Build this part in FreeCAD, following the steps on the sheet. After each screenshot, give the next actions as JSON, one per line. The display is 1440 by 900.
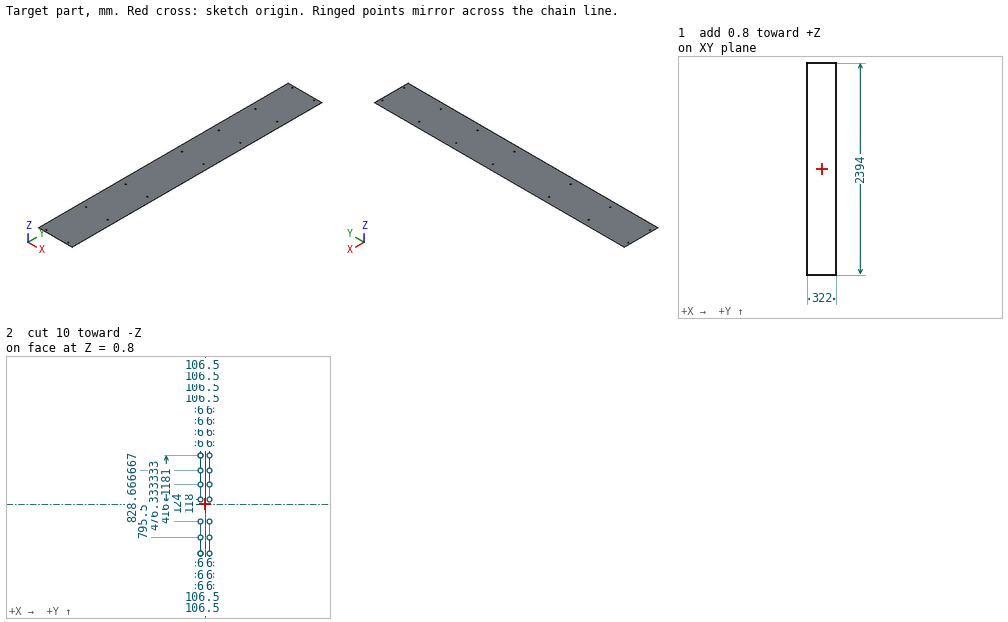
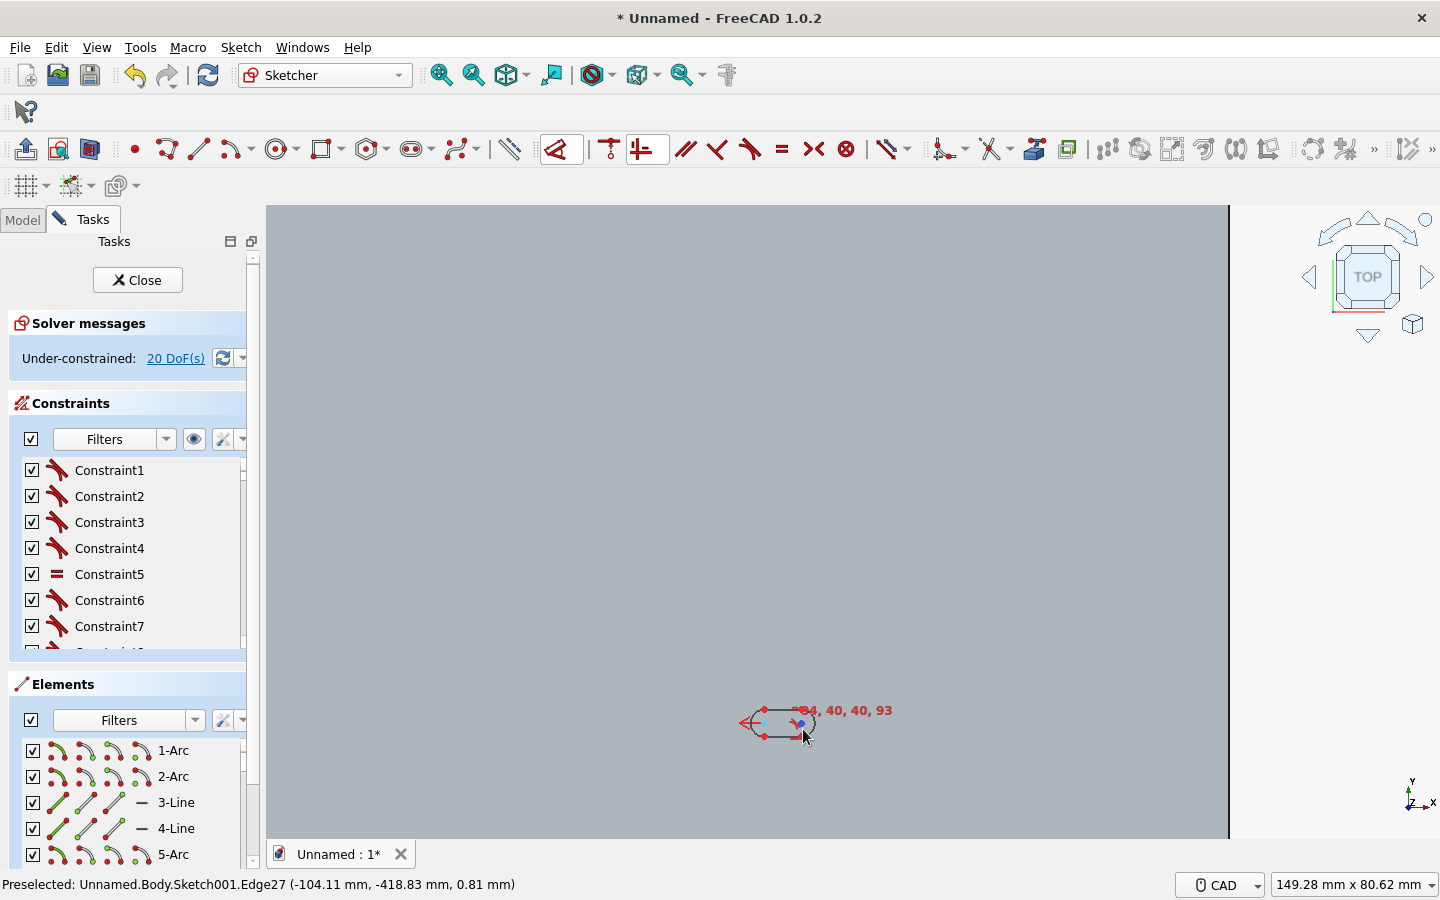
{"action": "left_click", "coordinate": [775, 710]}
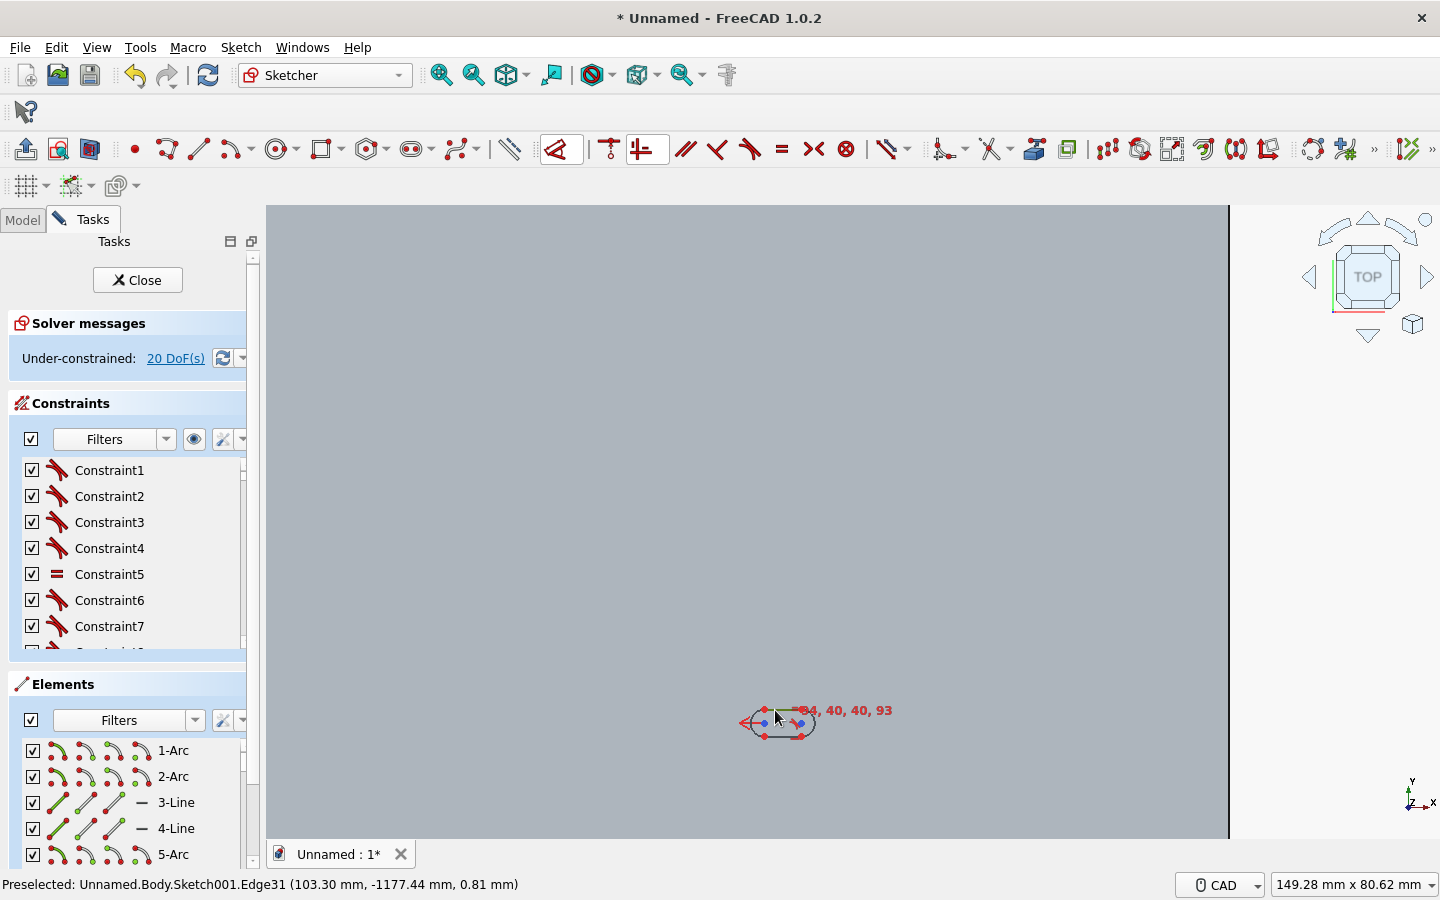
{"action": "key", "text": "l"}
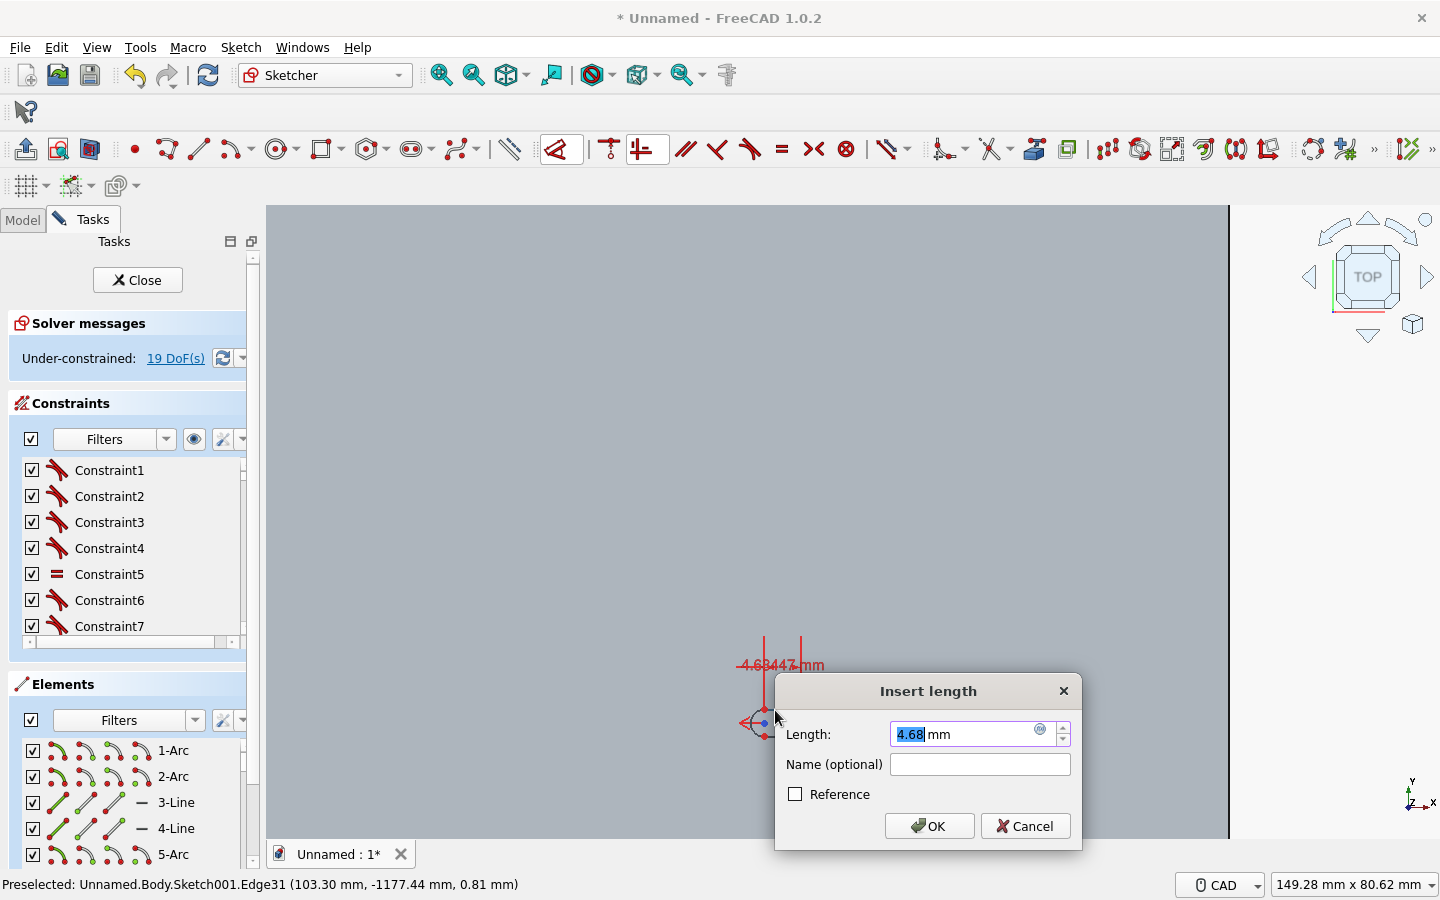
{"action": "type", "text": "6"}
{"action": "key", "text": "Return"}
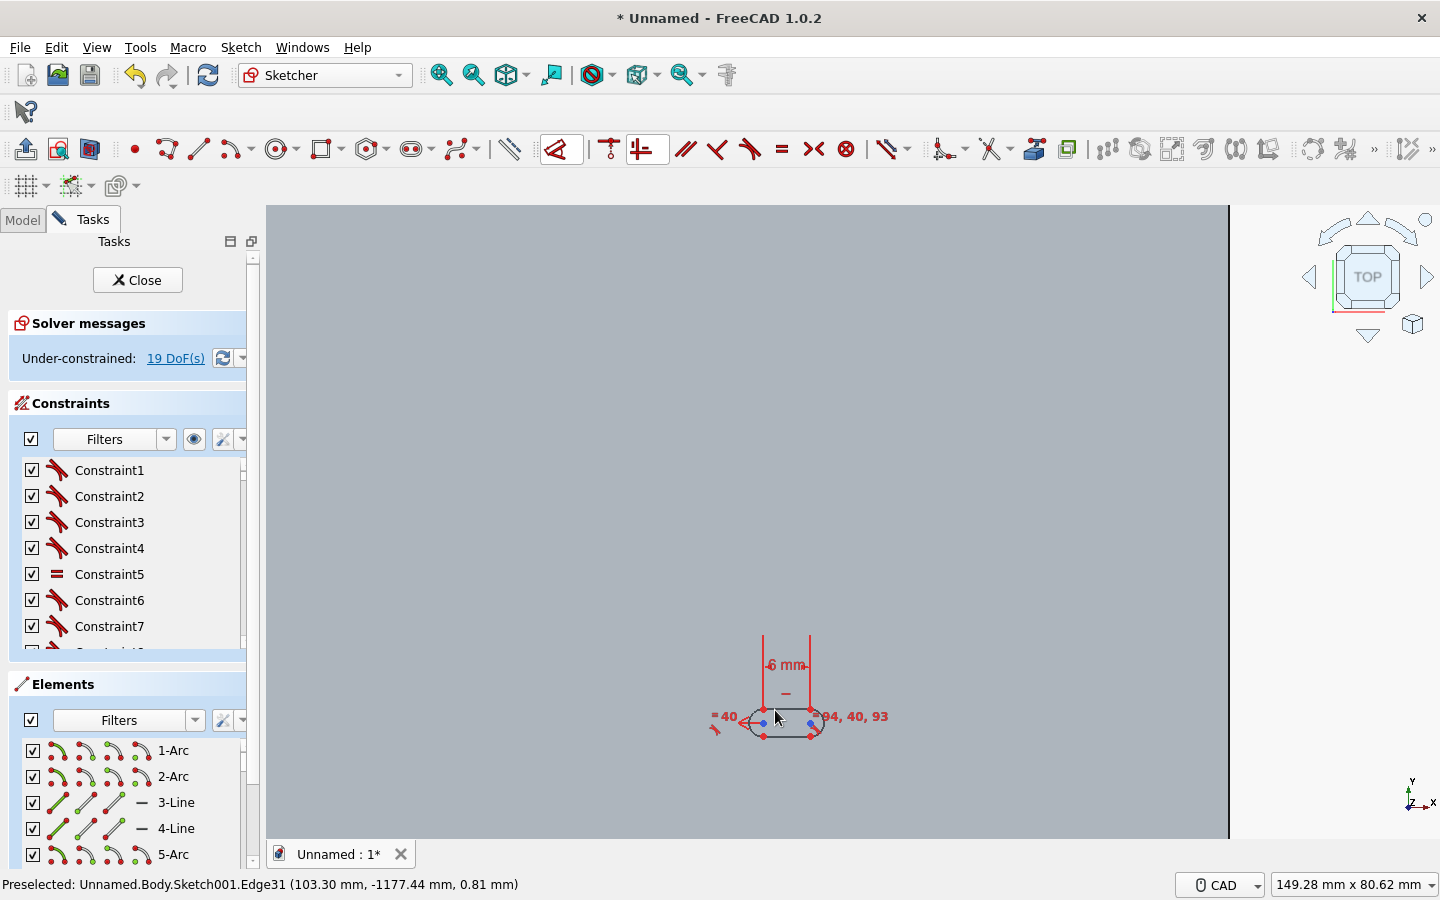
{"action": "scroll", "coordinate": [808, 777], "scroll_direction": "down", "scroll_amount": 18}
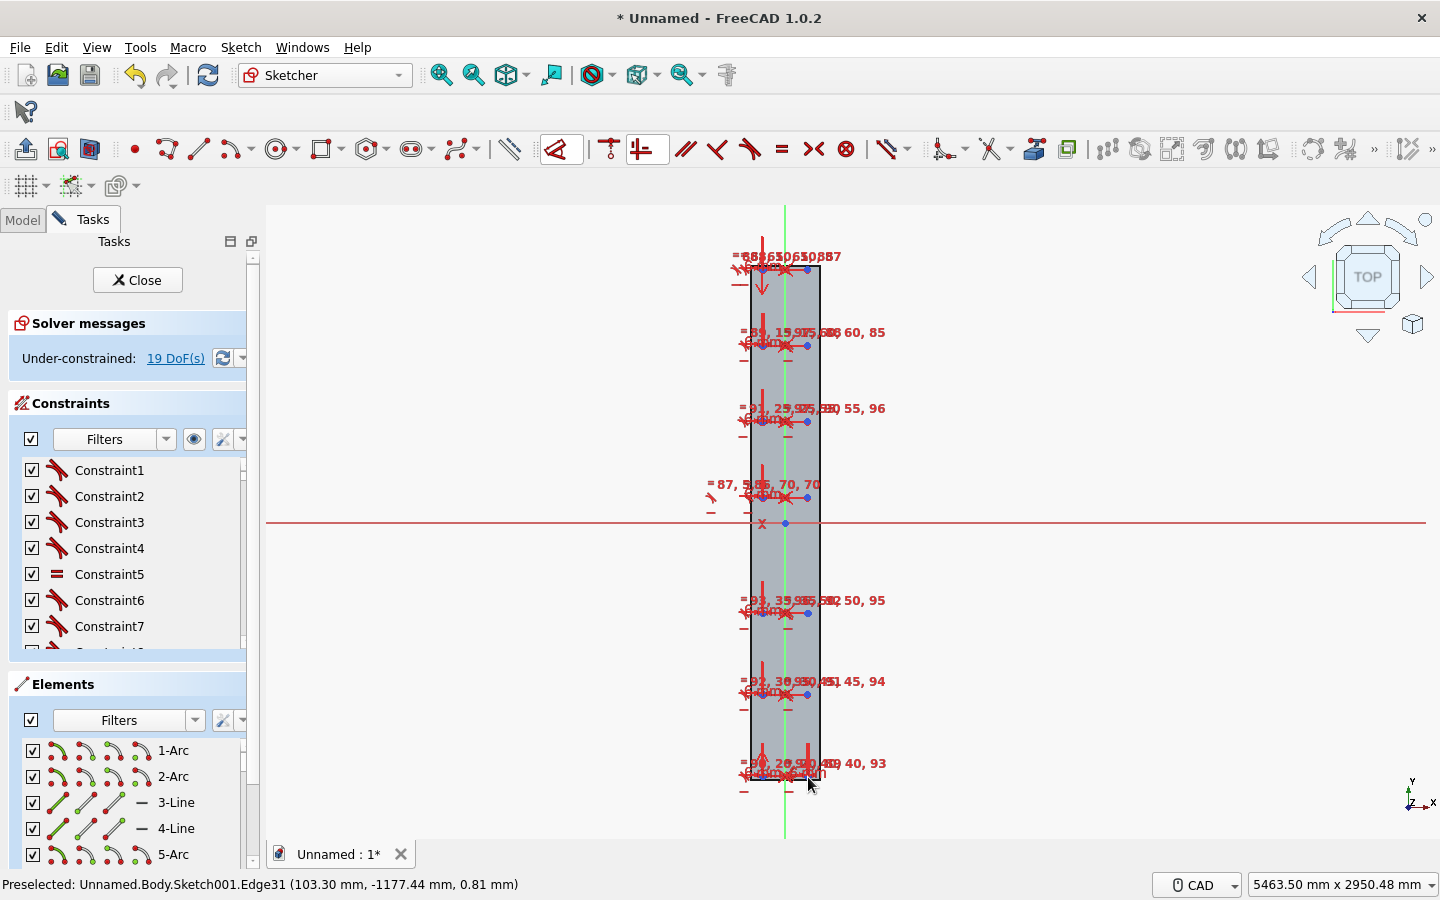
{"action": "scroll", "coordinate": [808, 694], "scroll_direction": "up", "scroll_amount": 18}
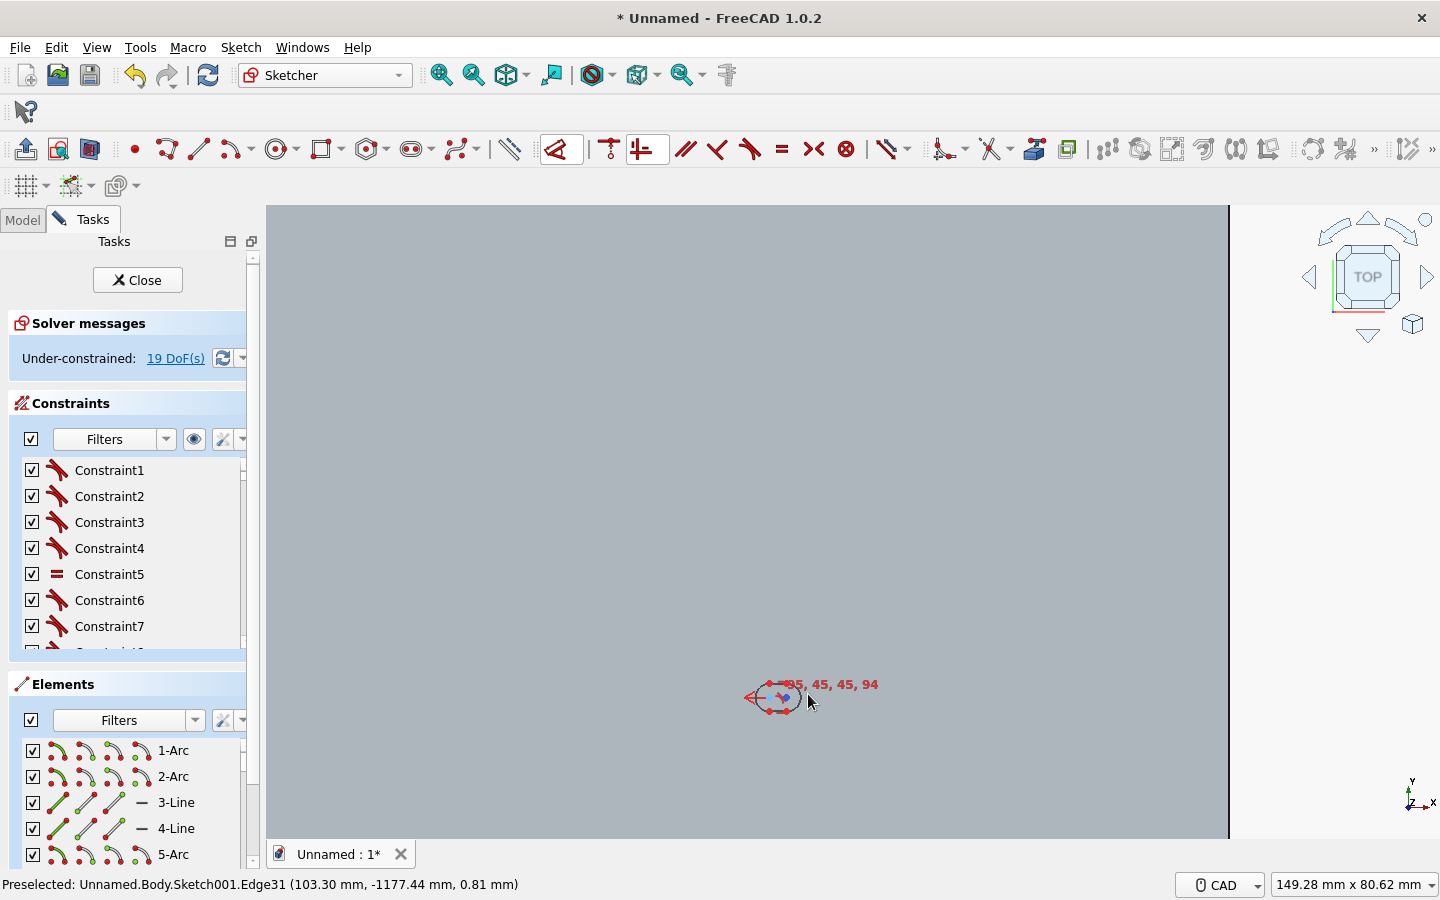
{"action": "scroll", "coordinate": [778, 684], "scroll_direction": "up", "scroll_amount": 4}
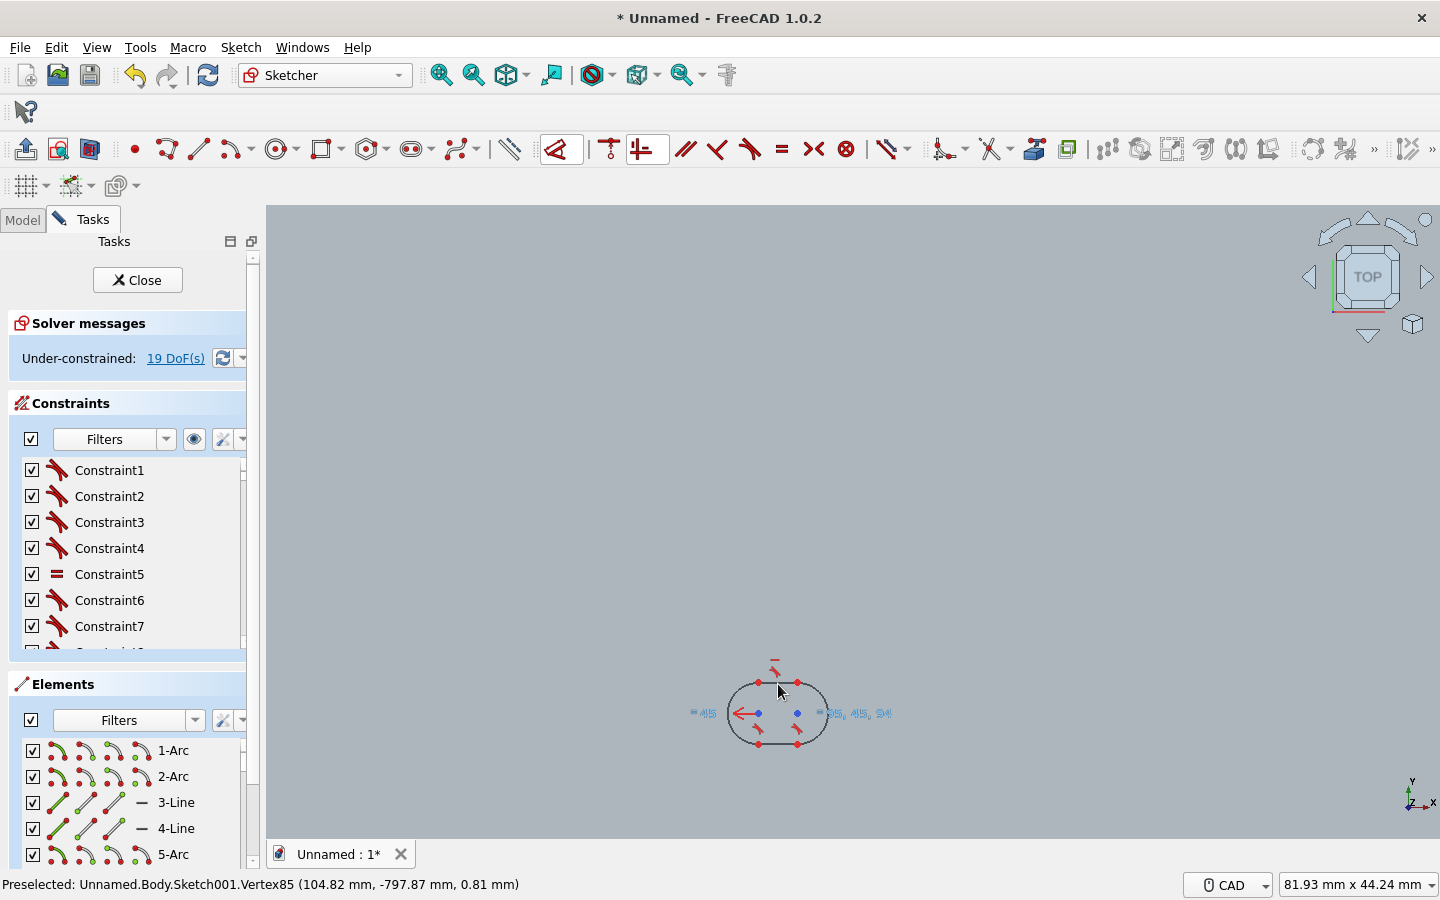
{"action": "left_click", "coordinate": [778, 683]}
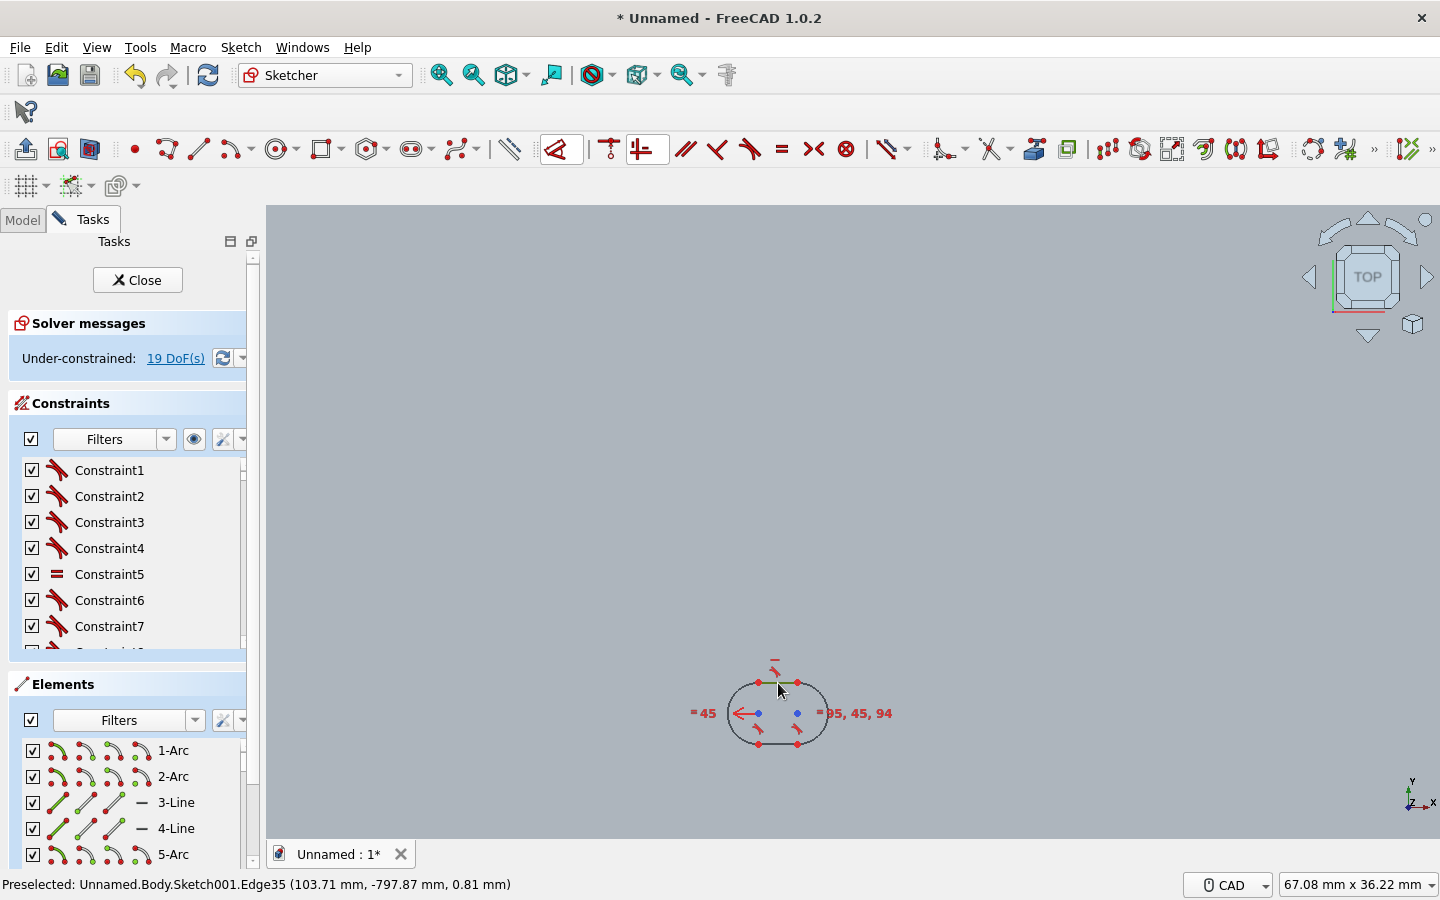
{"action": "key", "text": "l"}